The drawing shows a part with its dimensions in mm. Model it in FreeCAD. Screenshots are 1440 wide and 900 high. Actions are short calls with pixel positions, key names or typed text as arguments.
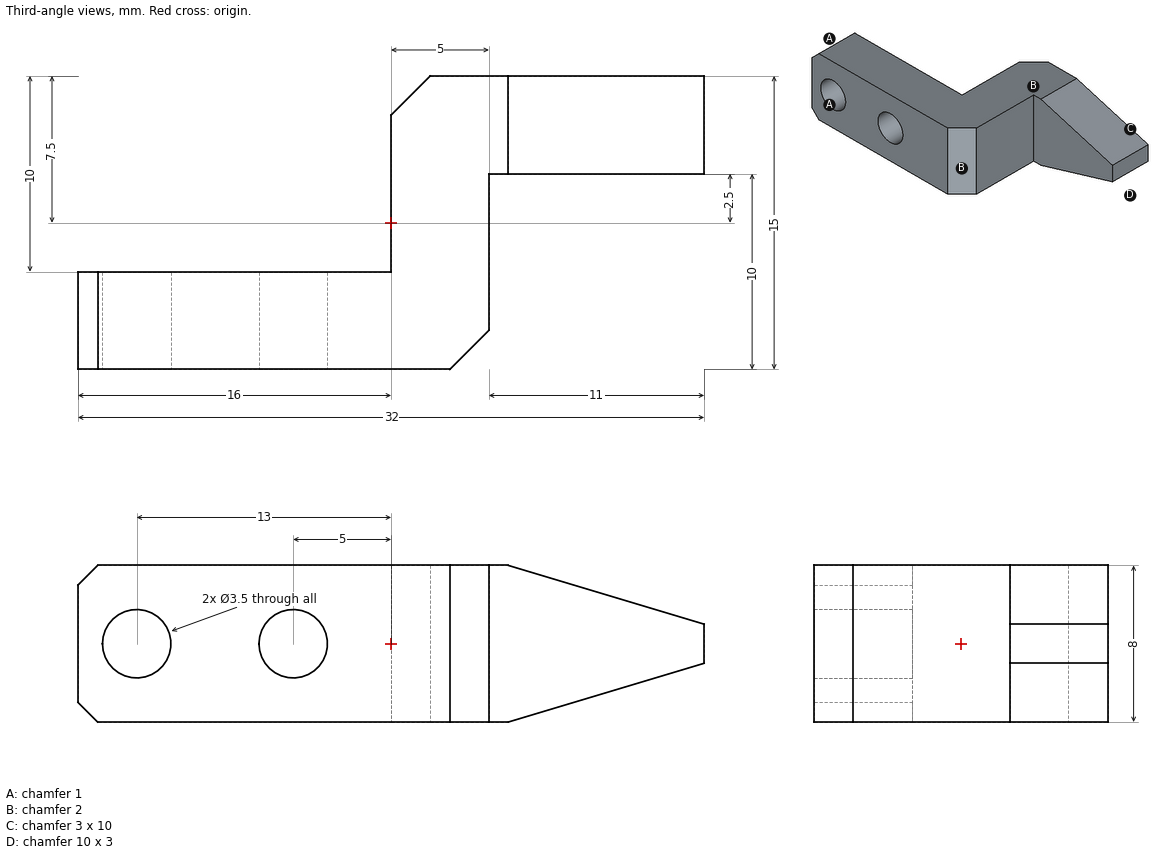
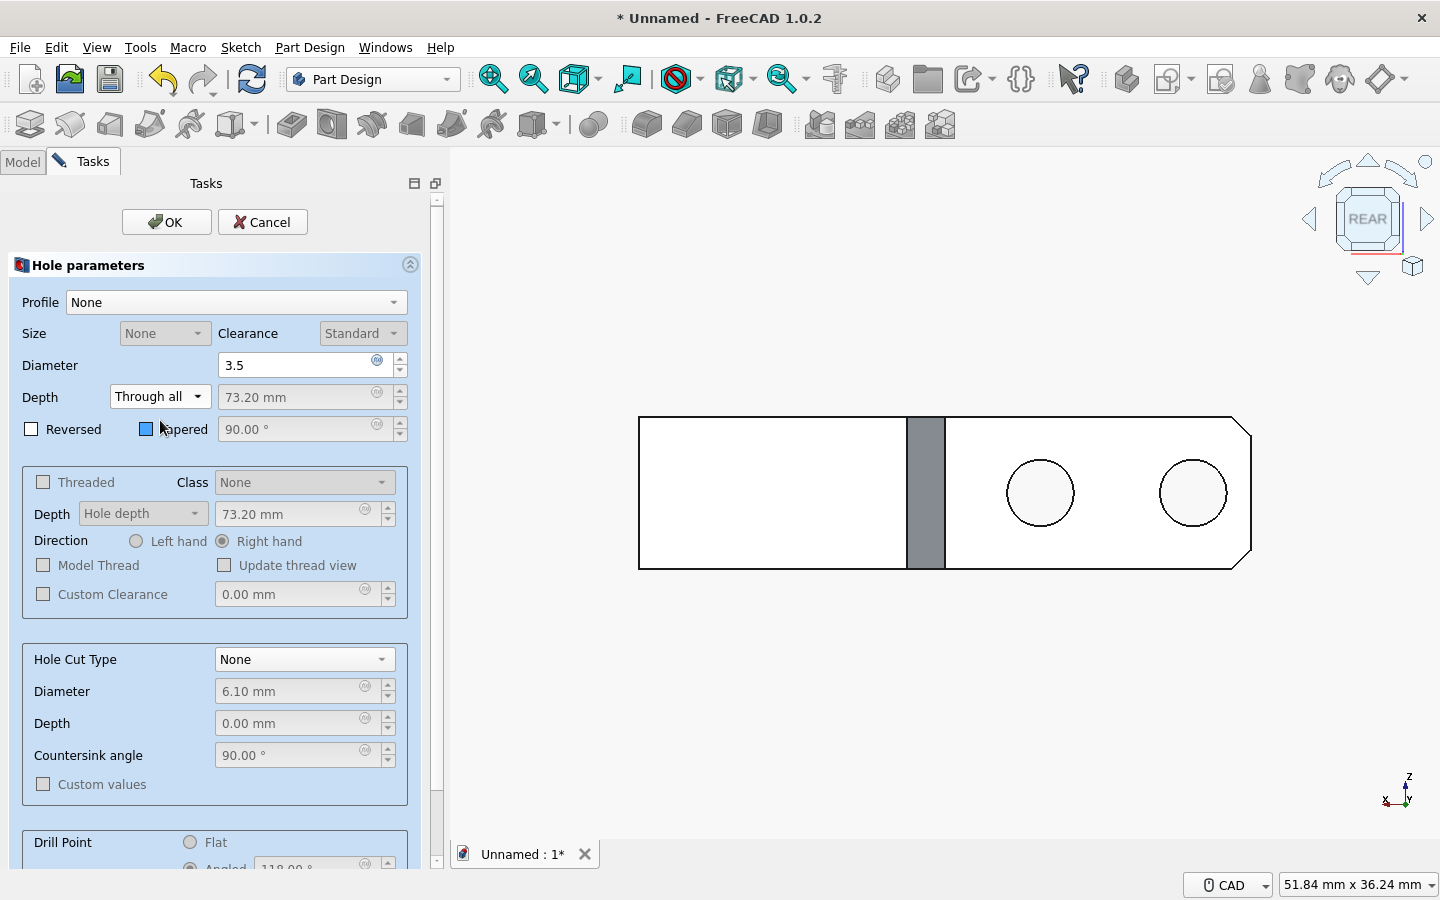
click(167, 222)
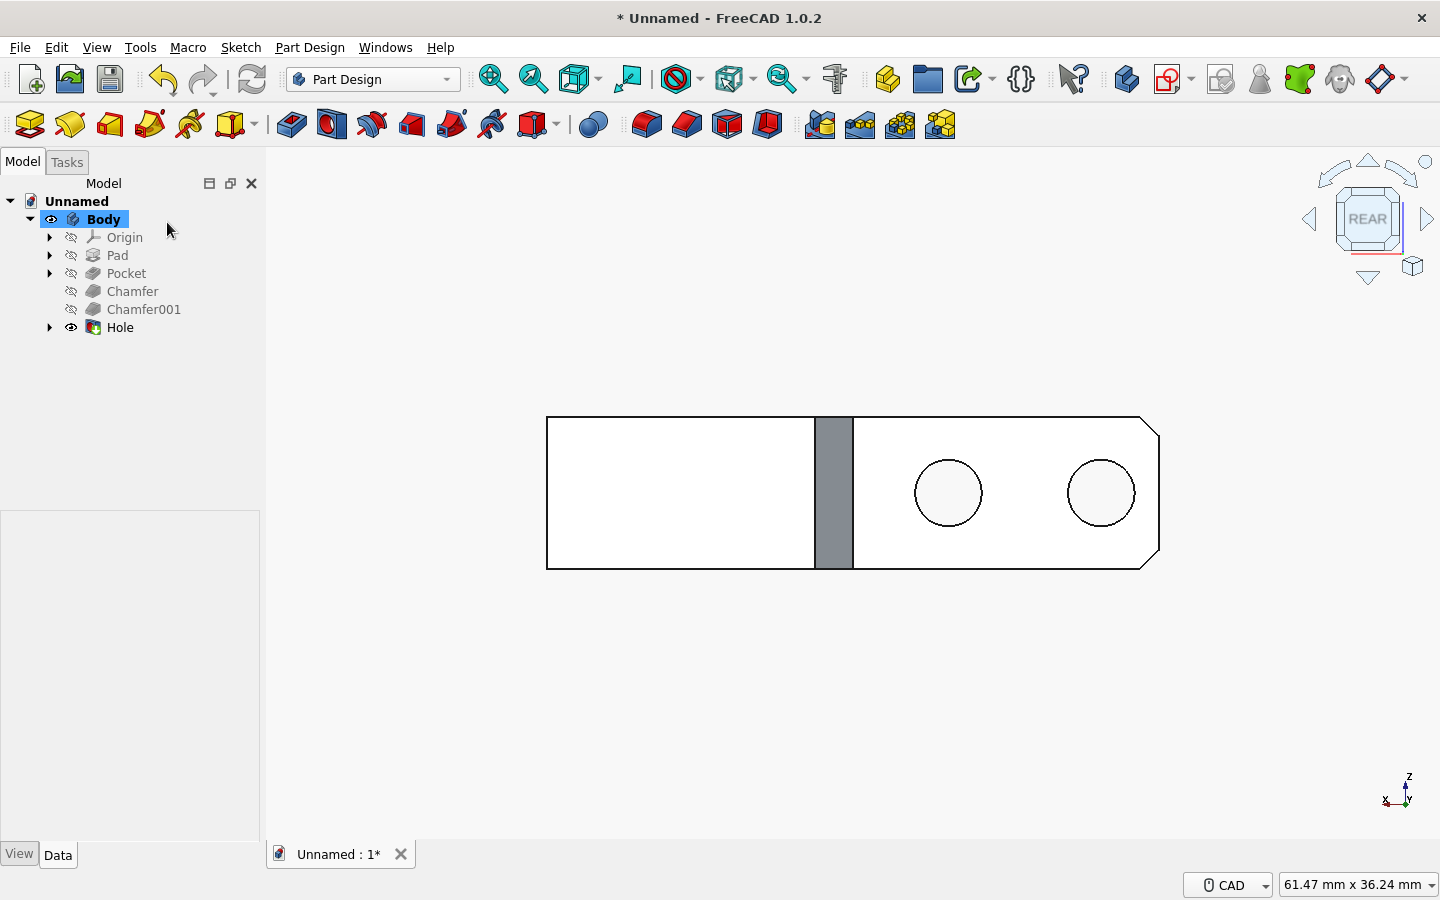
key(0)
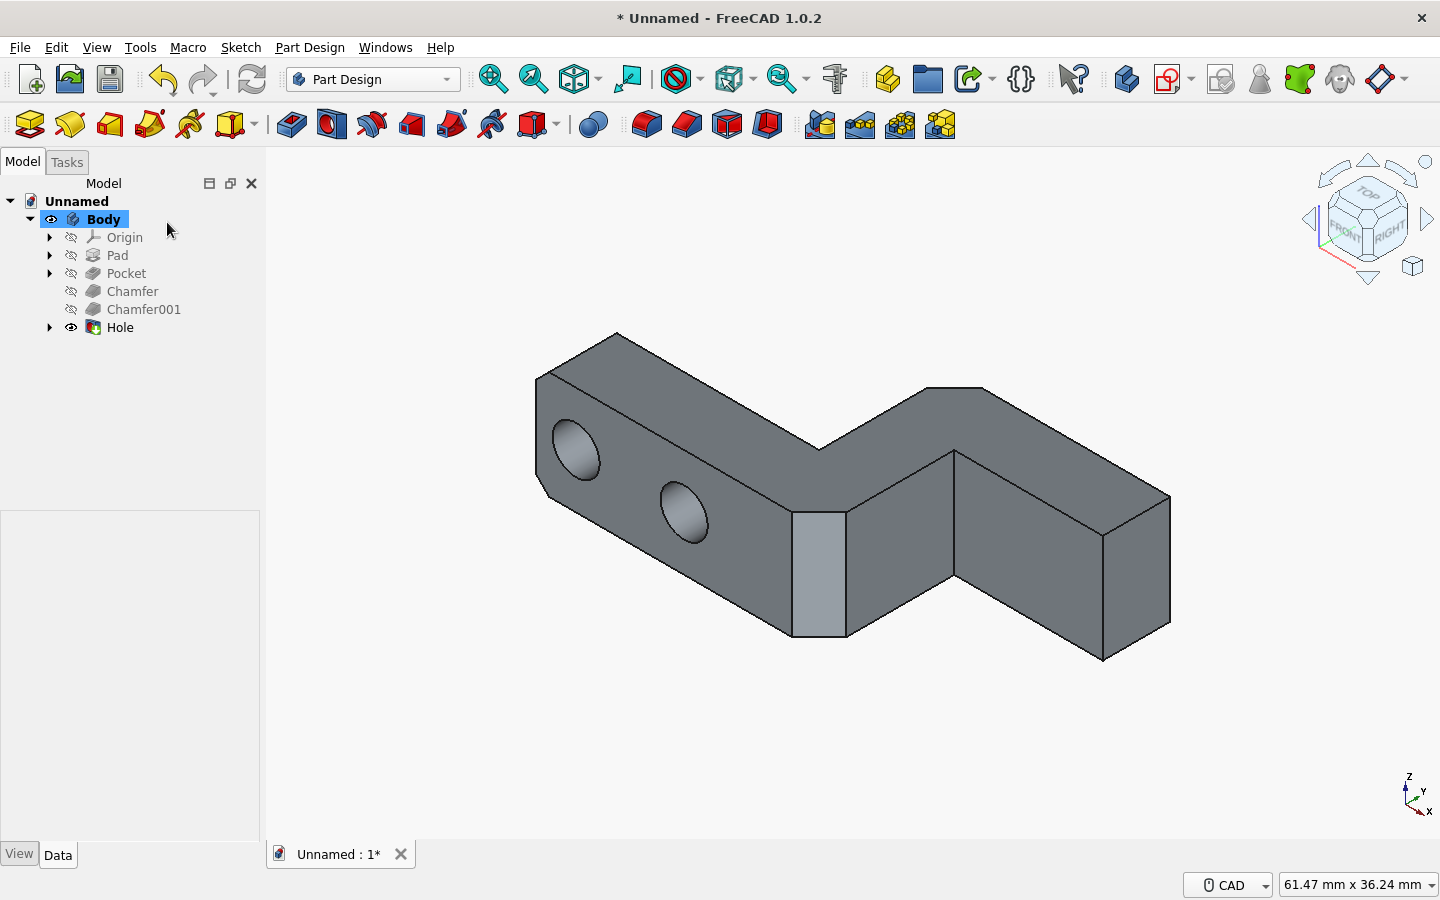
click(1137, 515)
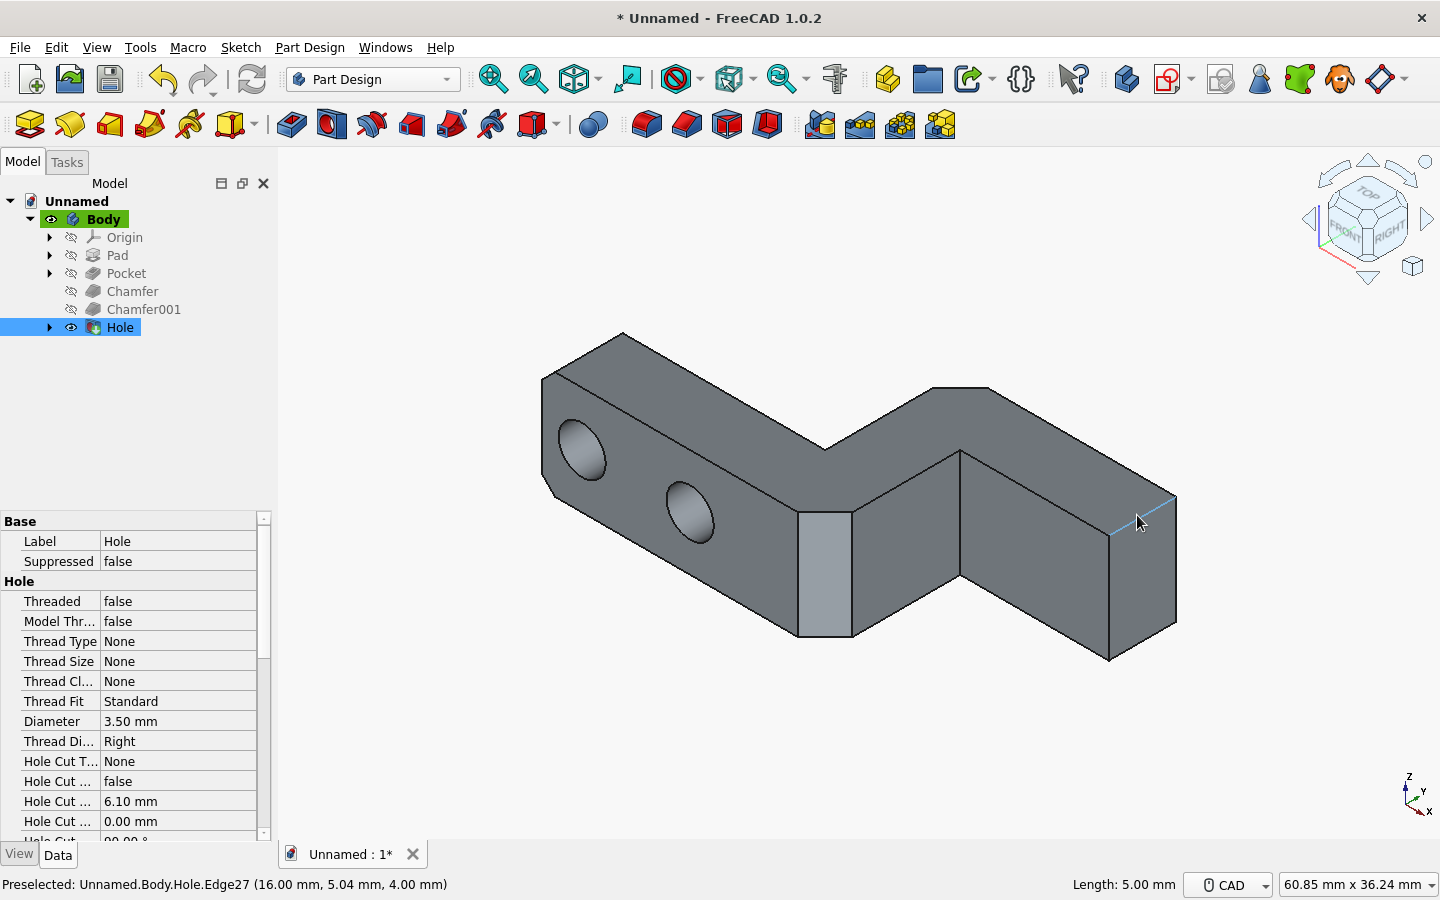
click(688, 124)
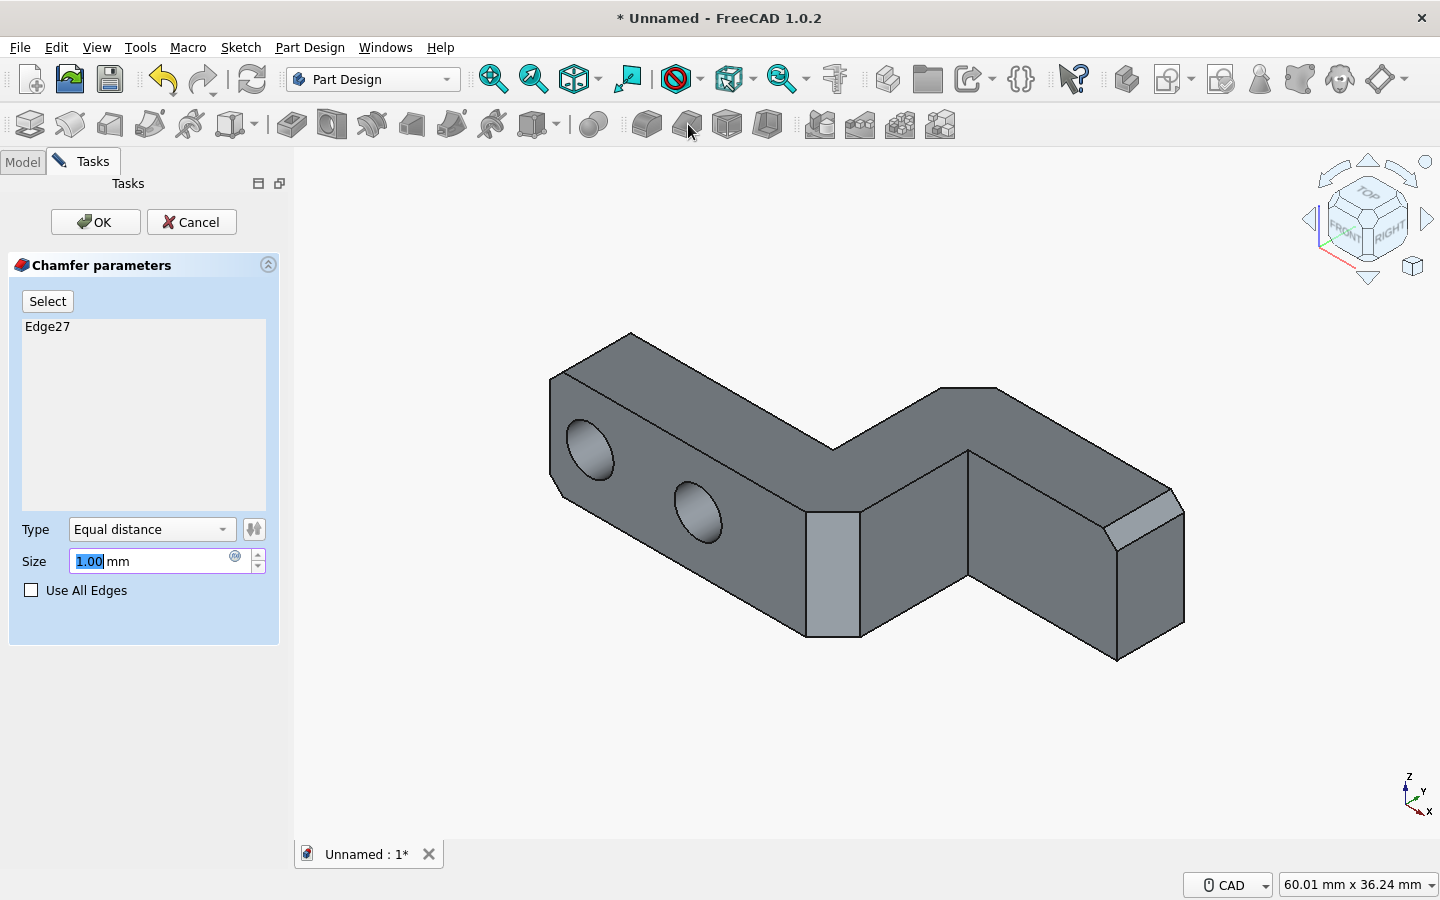
text(3)
key(Tab)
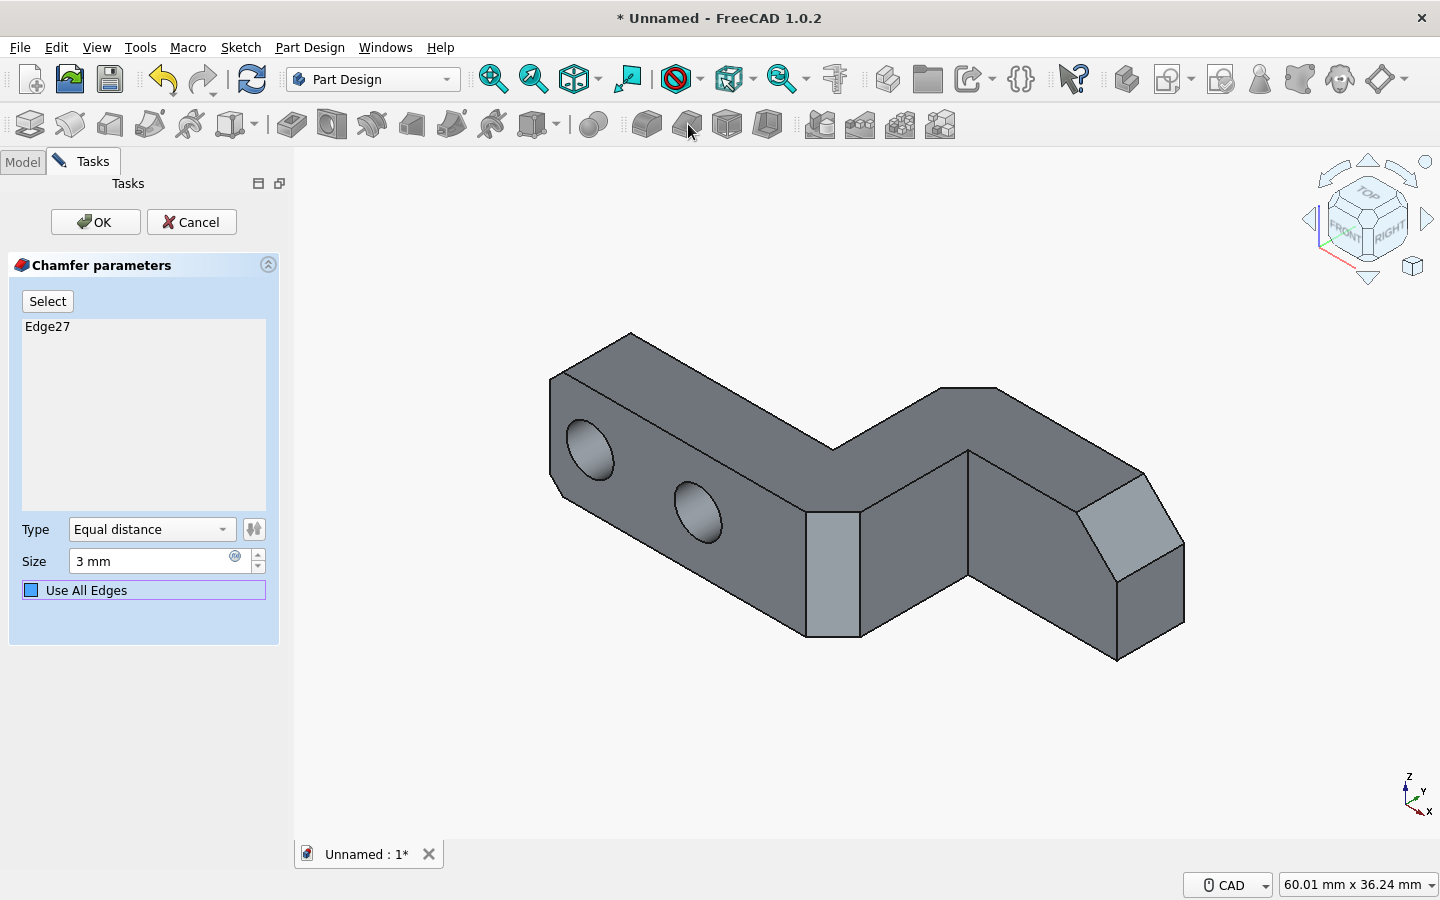
click(153, 530)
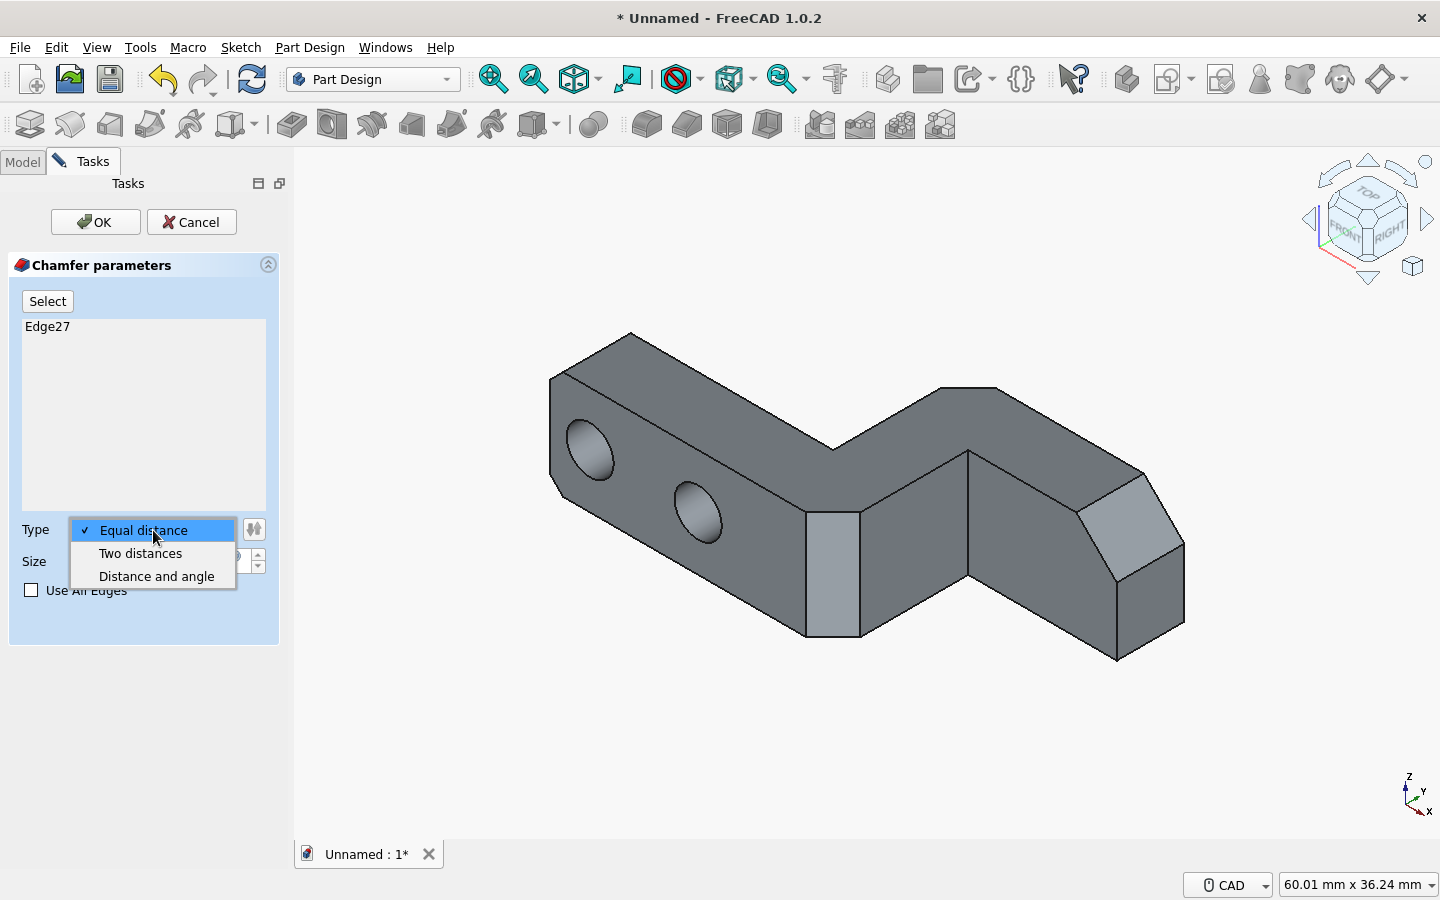
click(152, 554)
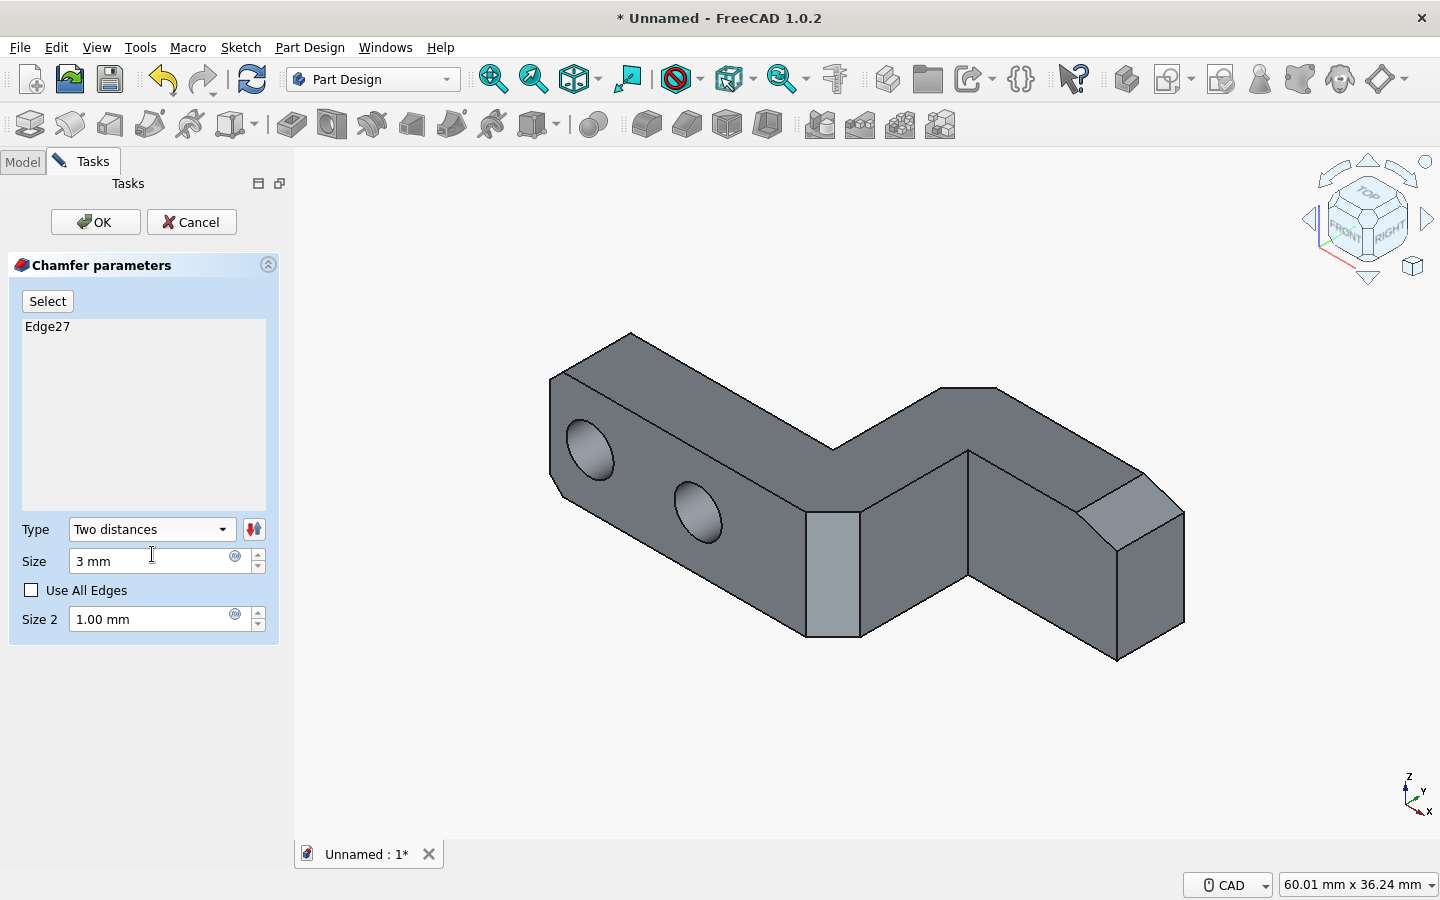
triple_click(160, 619)